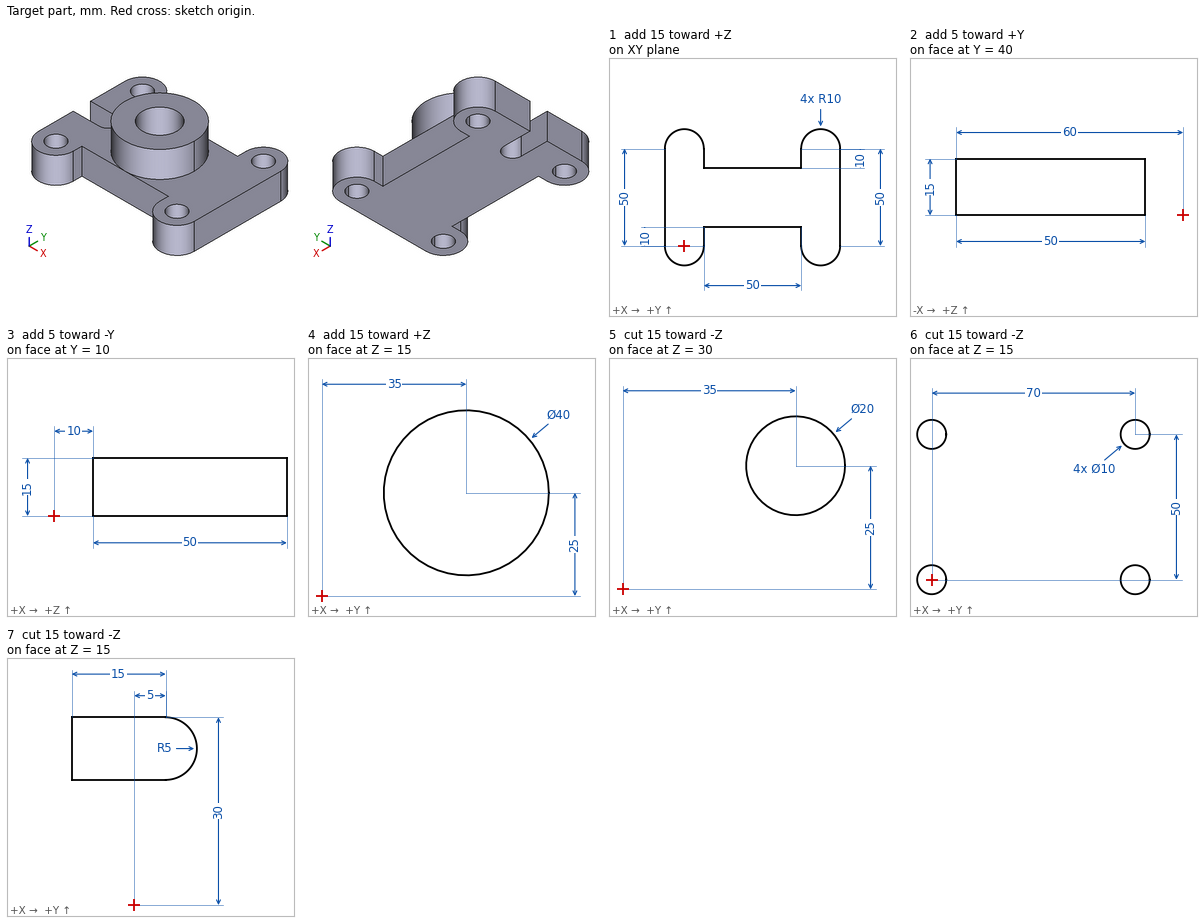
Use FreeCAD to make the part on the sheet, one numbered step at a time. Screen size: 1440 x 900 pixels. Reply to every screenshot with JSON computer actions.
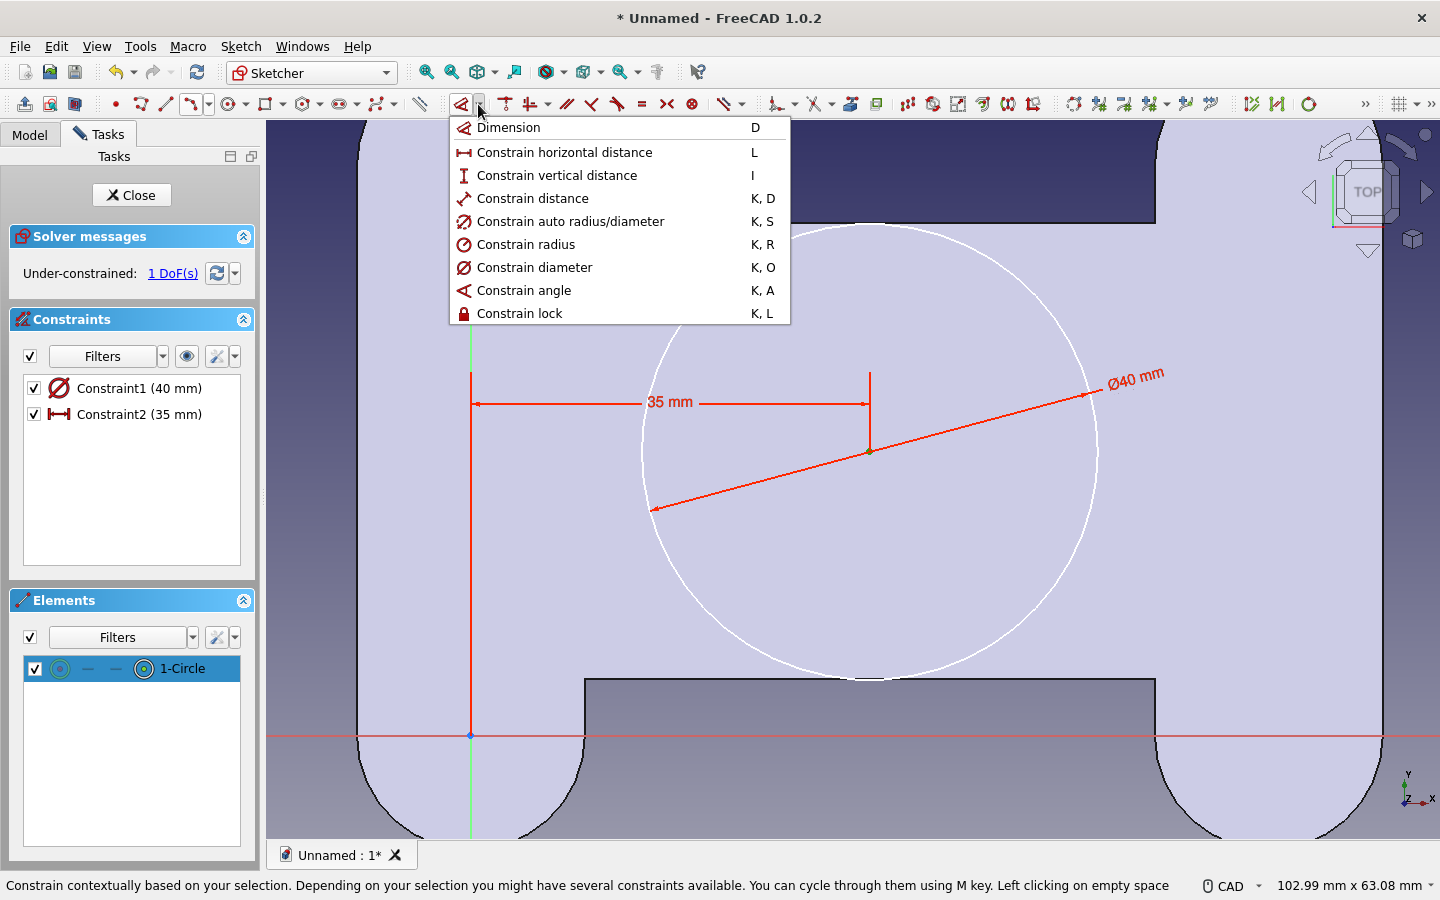
{"action": "left_click", "coordinate": [620, 176]}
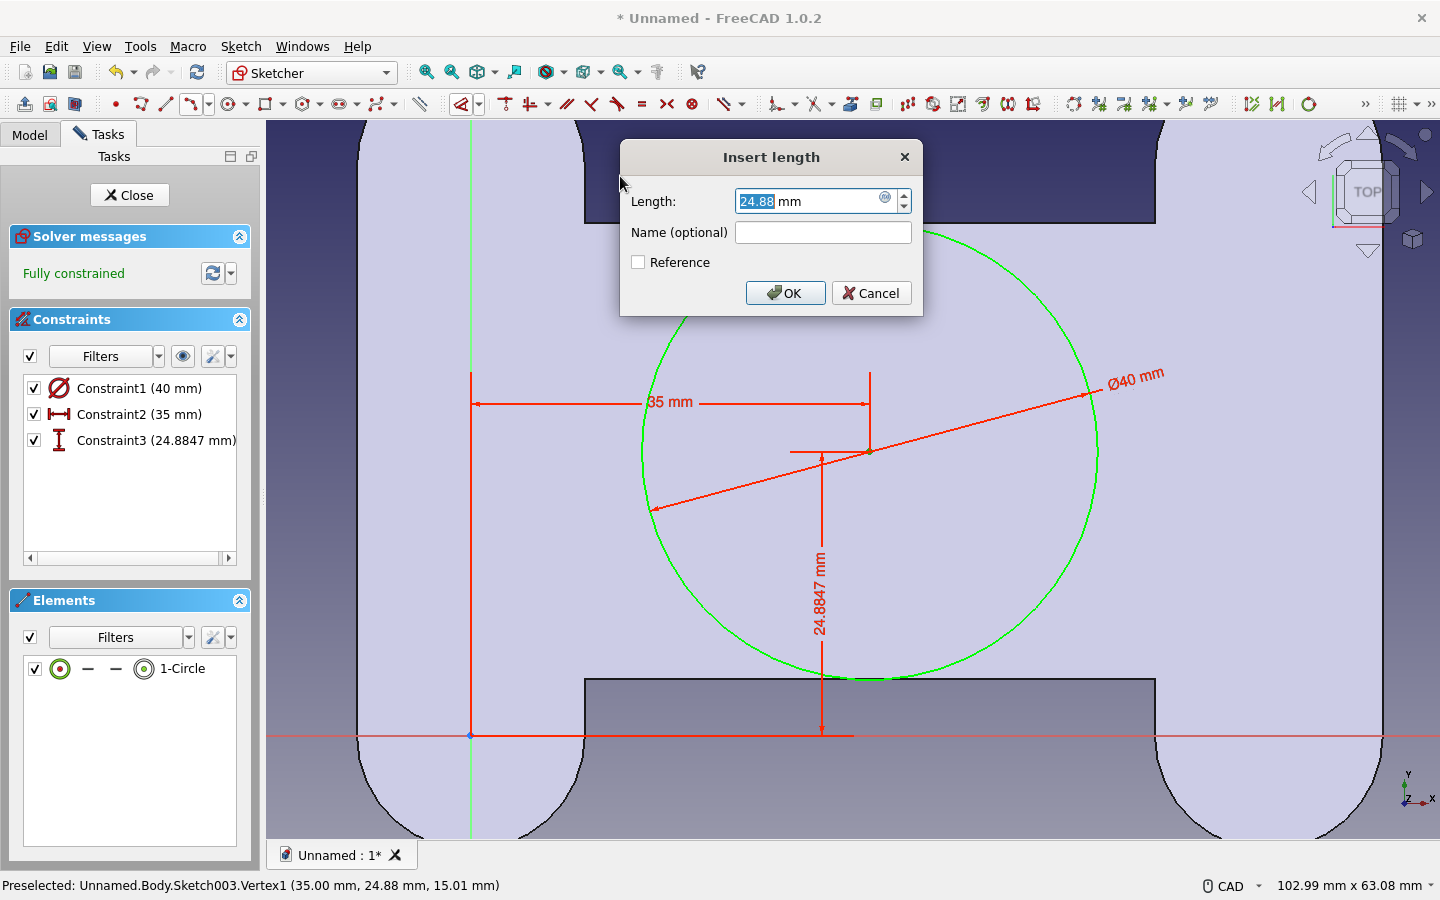
{"action": "type", "text": "25"}
{"action": "key", "text": "Return"}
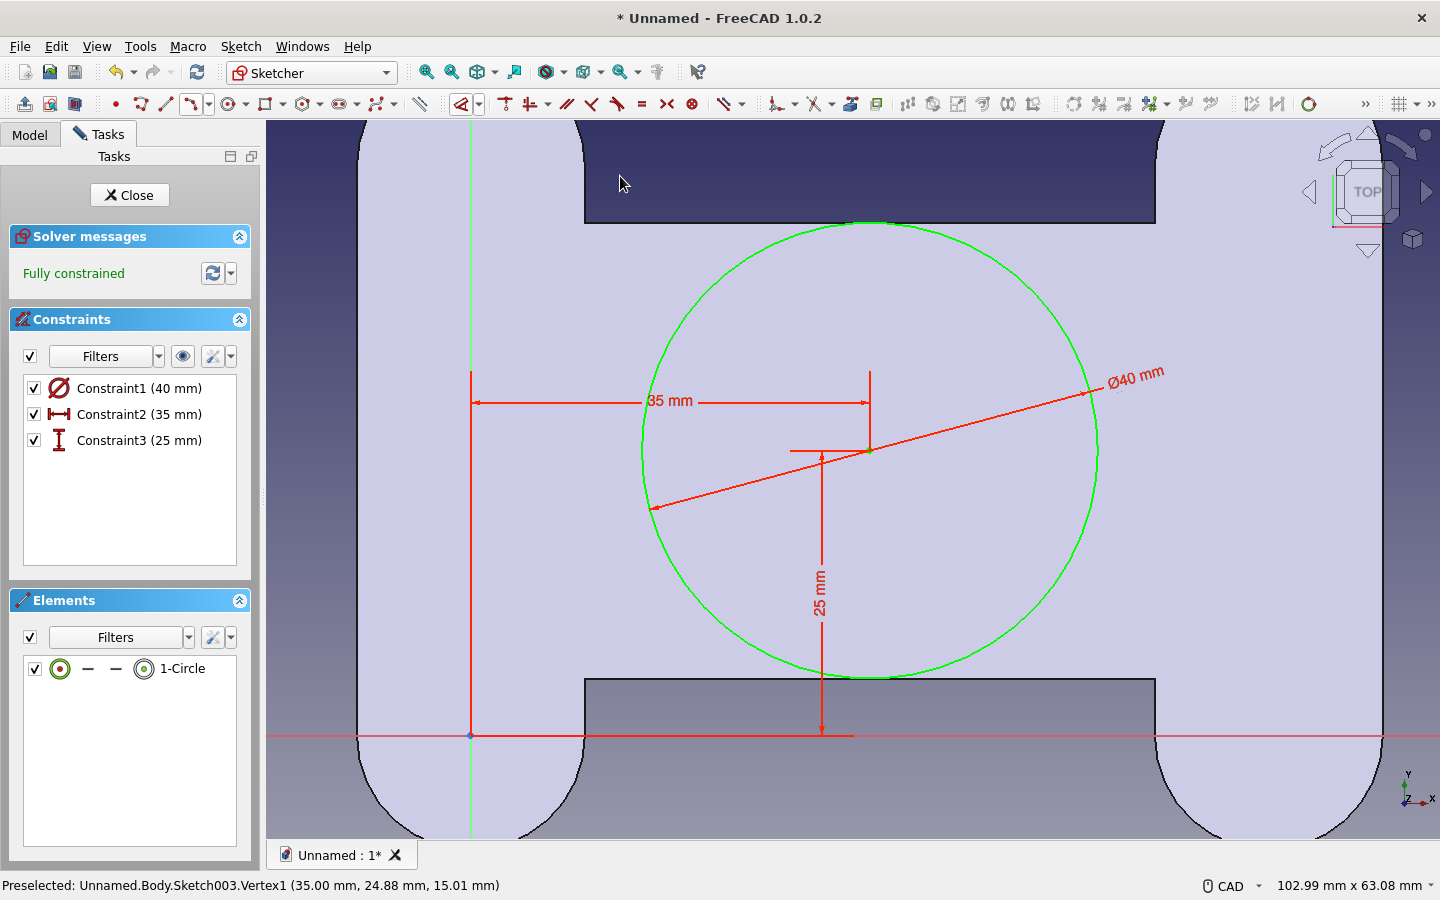
{"action": "left_click", "coordinate": [130, 195]}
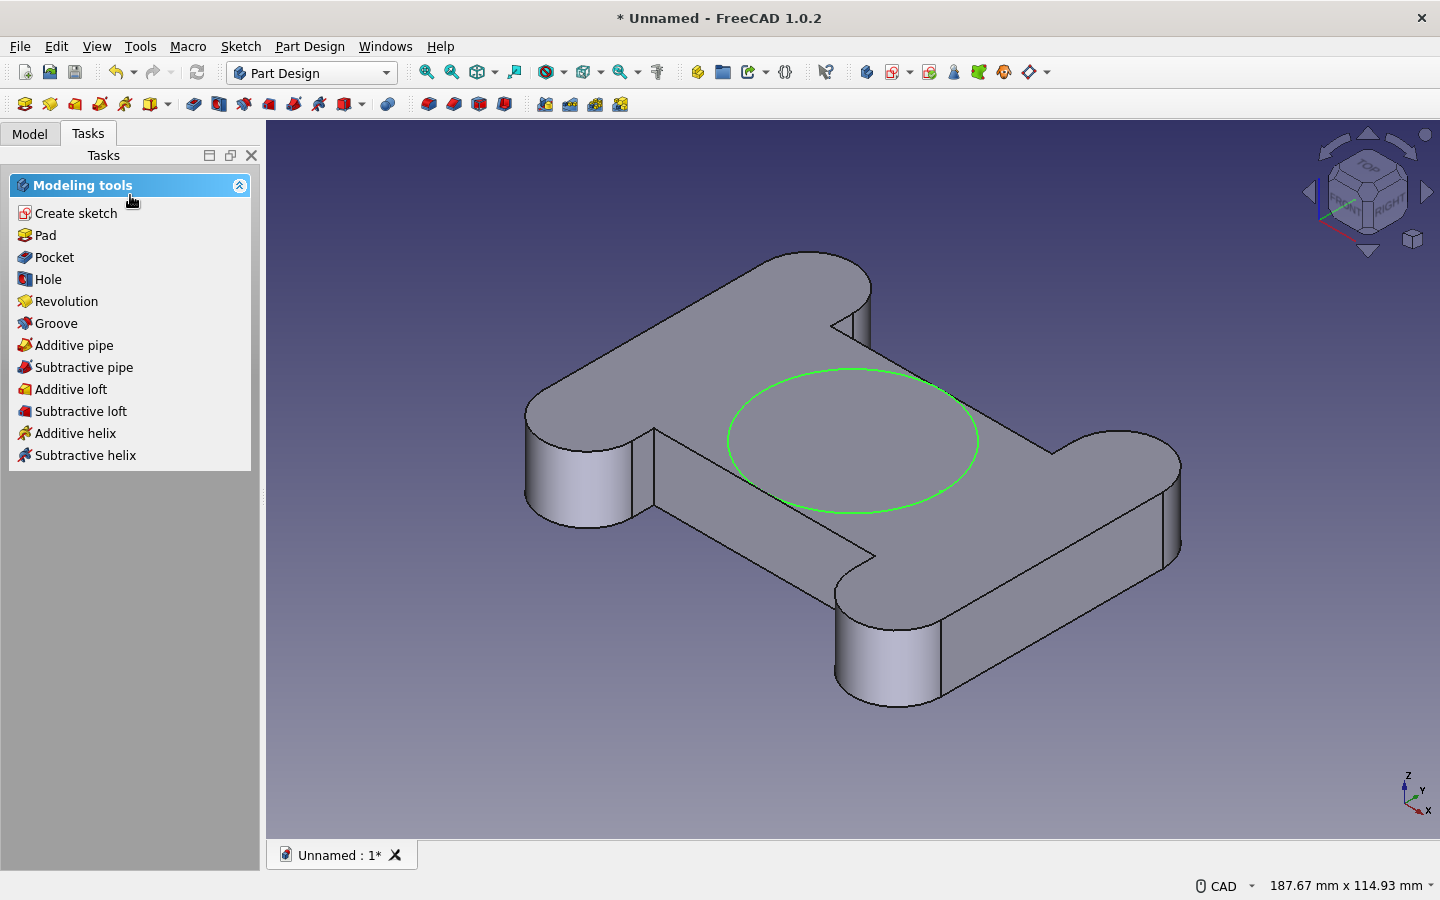
{"action": "left_click", "coordinate": [25, 104]}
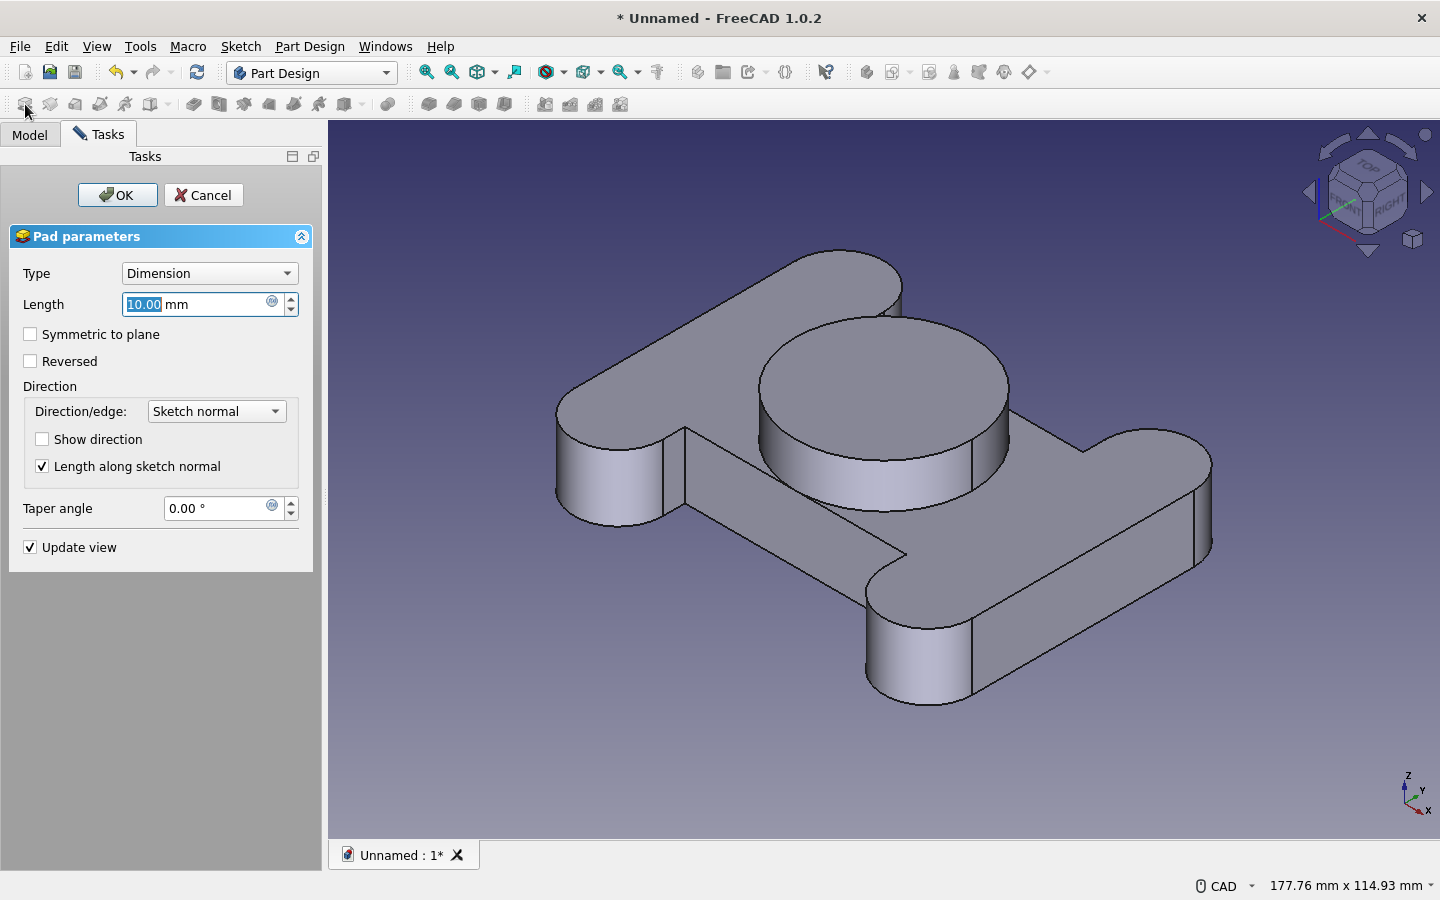
{"action": "type", "text": "15"}
{"action": "key", "text": "Tab"}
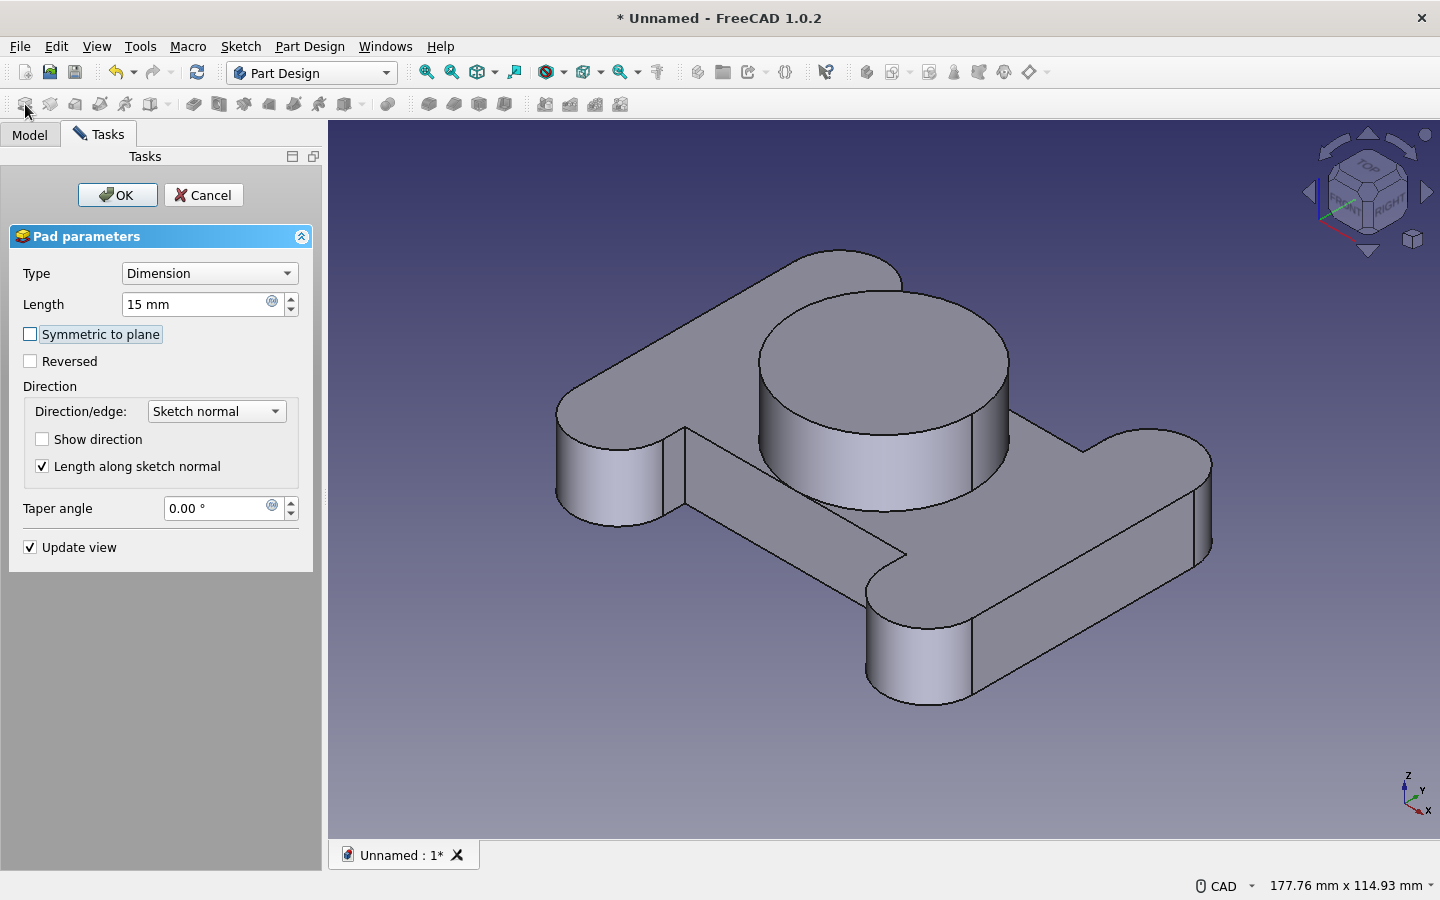
{"action": "left_click", "coordinate": [118, 195]}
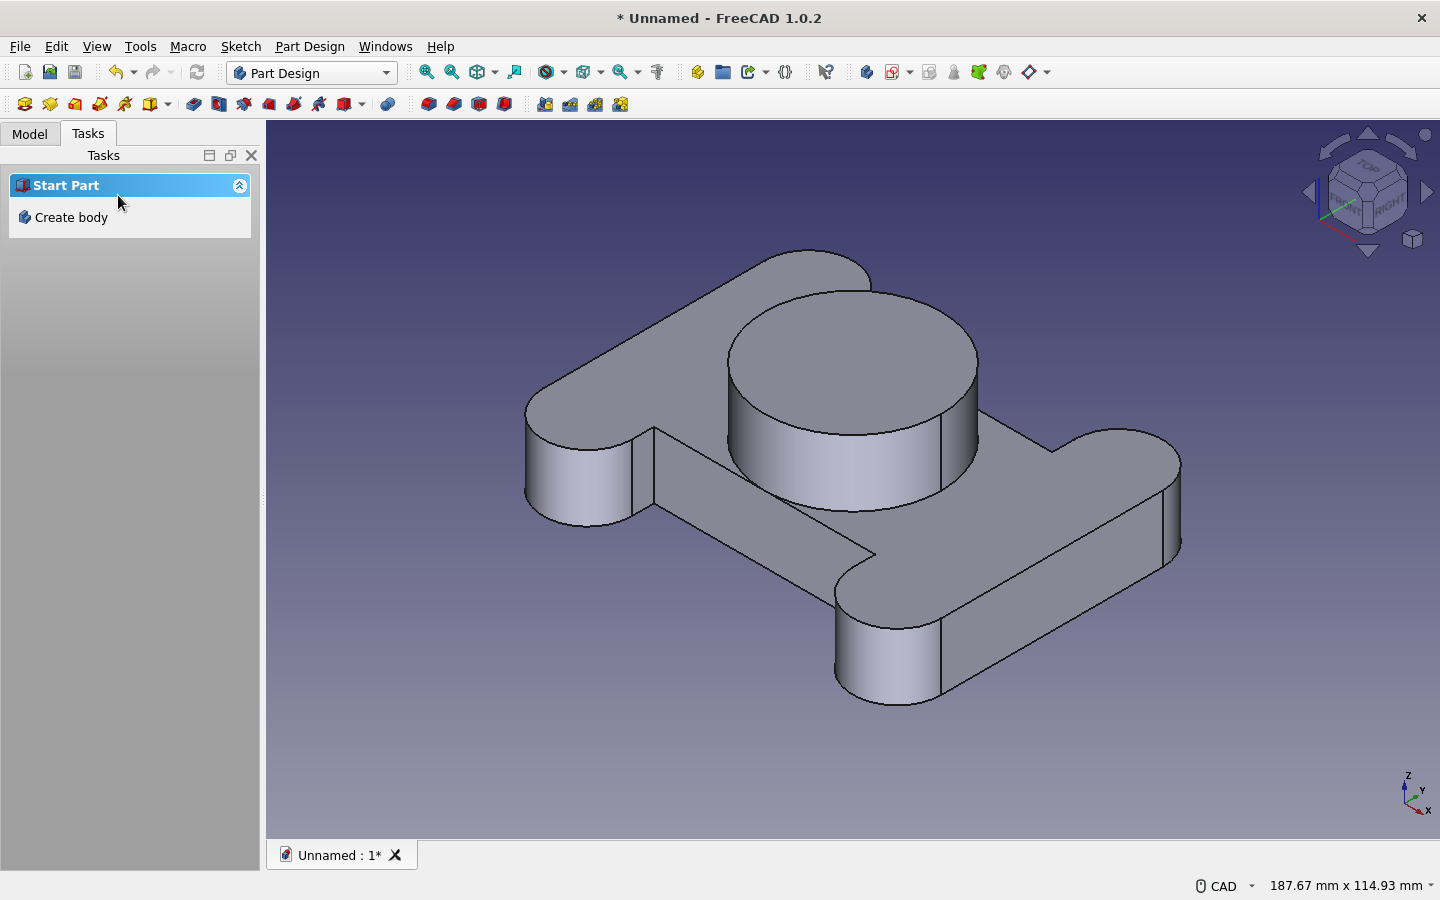
{"action": "left_click", "coordinate": [853, 362]}